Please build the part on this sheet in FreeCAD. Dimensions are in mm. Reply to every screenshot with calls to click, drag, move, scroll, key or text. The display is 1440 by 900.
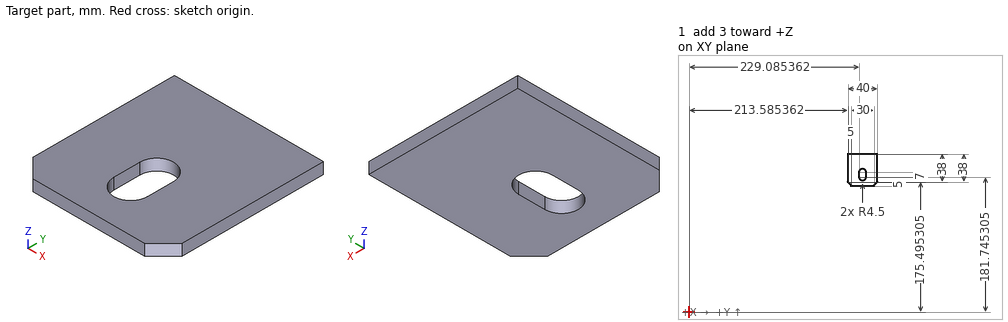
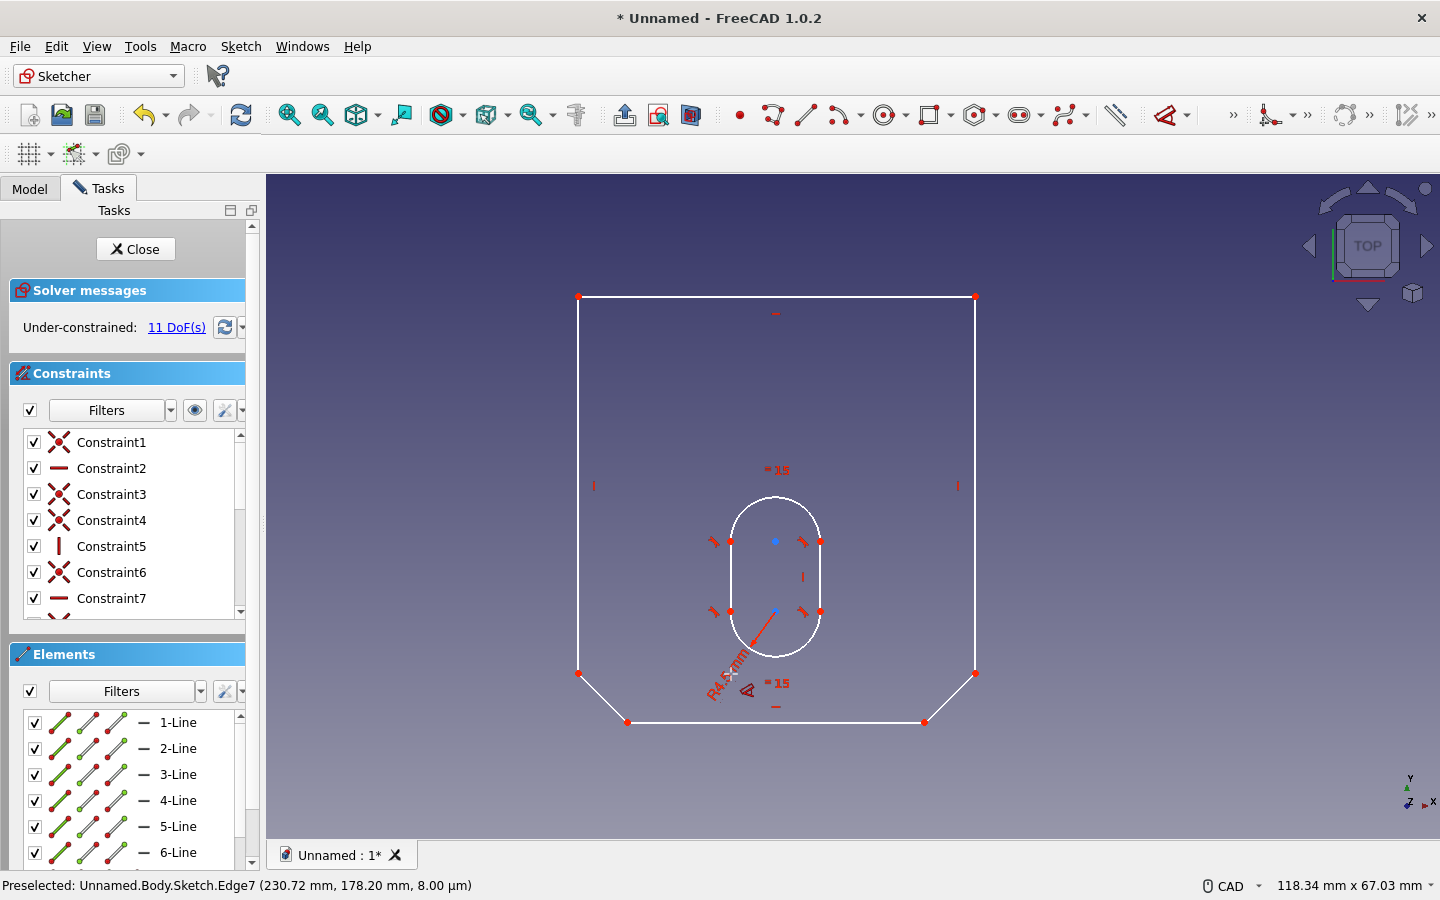
click(731, 591)
click(697, 577)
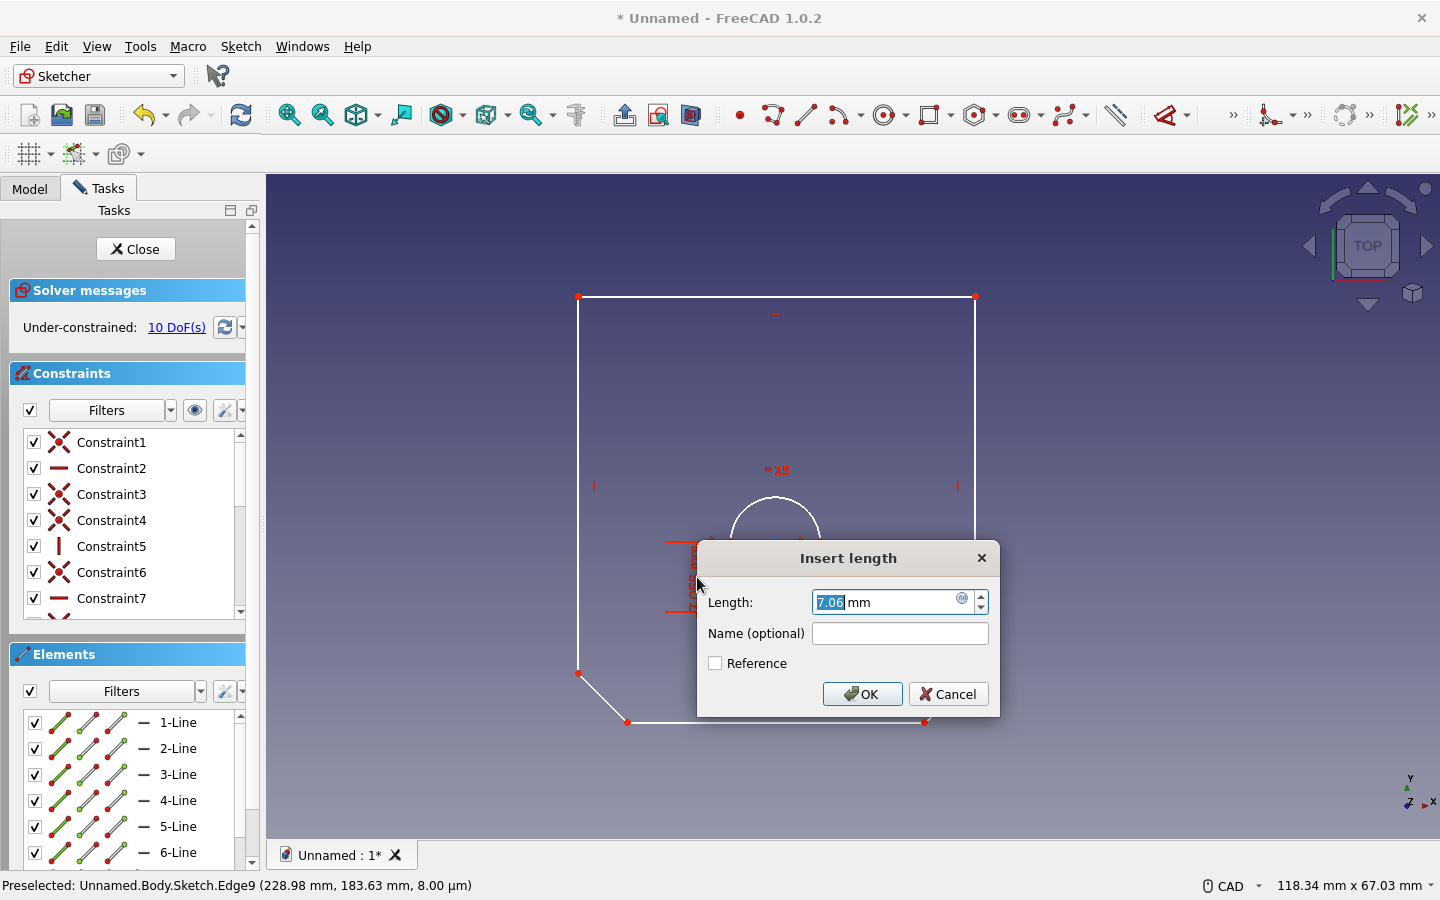
text(7)
key(Return)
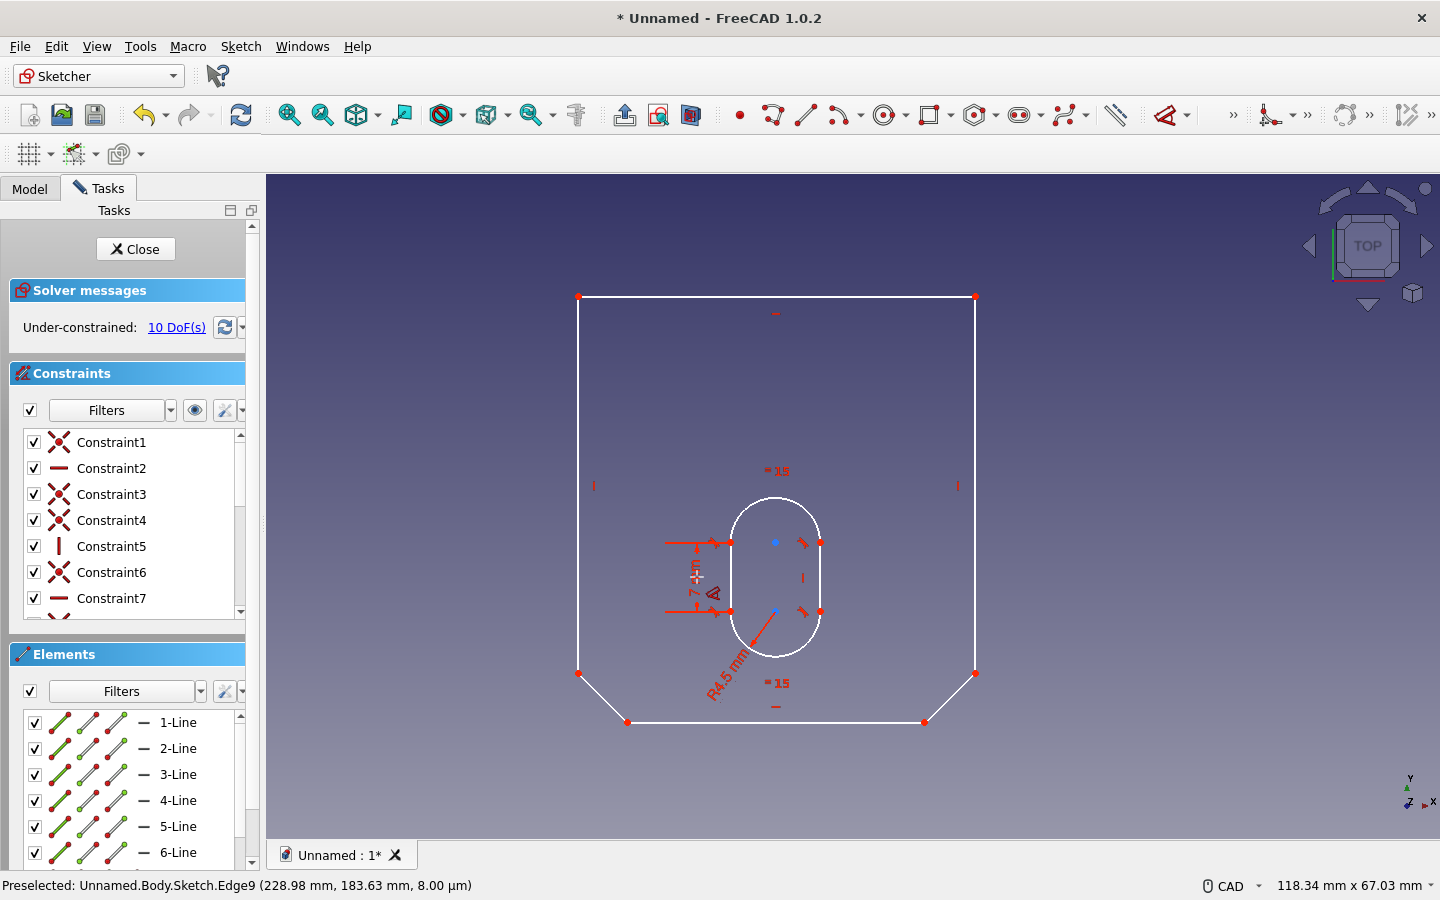
click(717, 723)
click(776, 757)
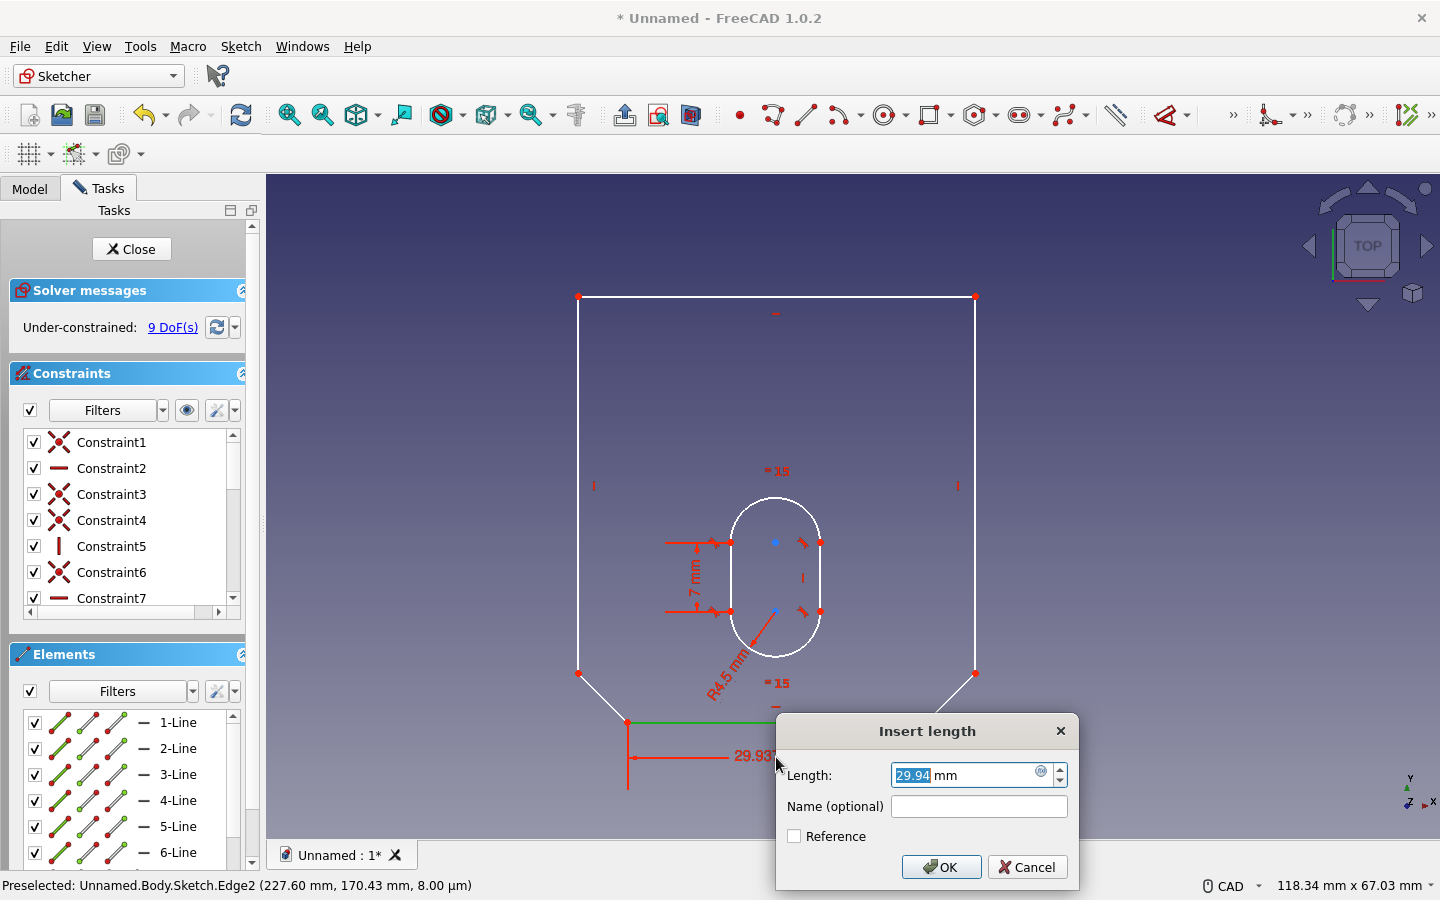
text(30)
key(Return)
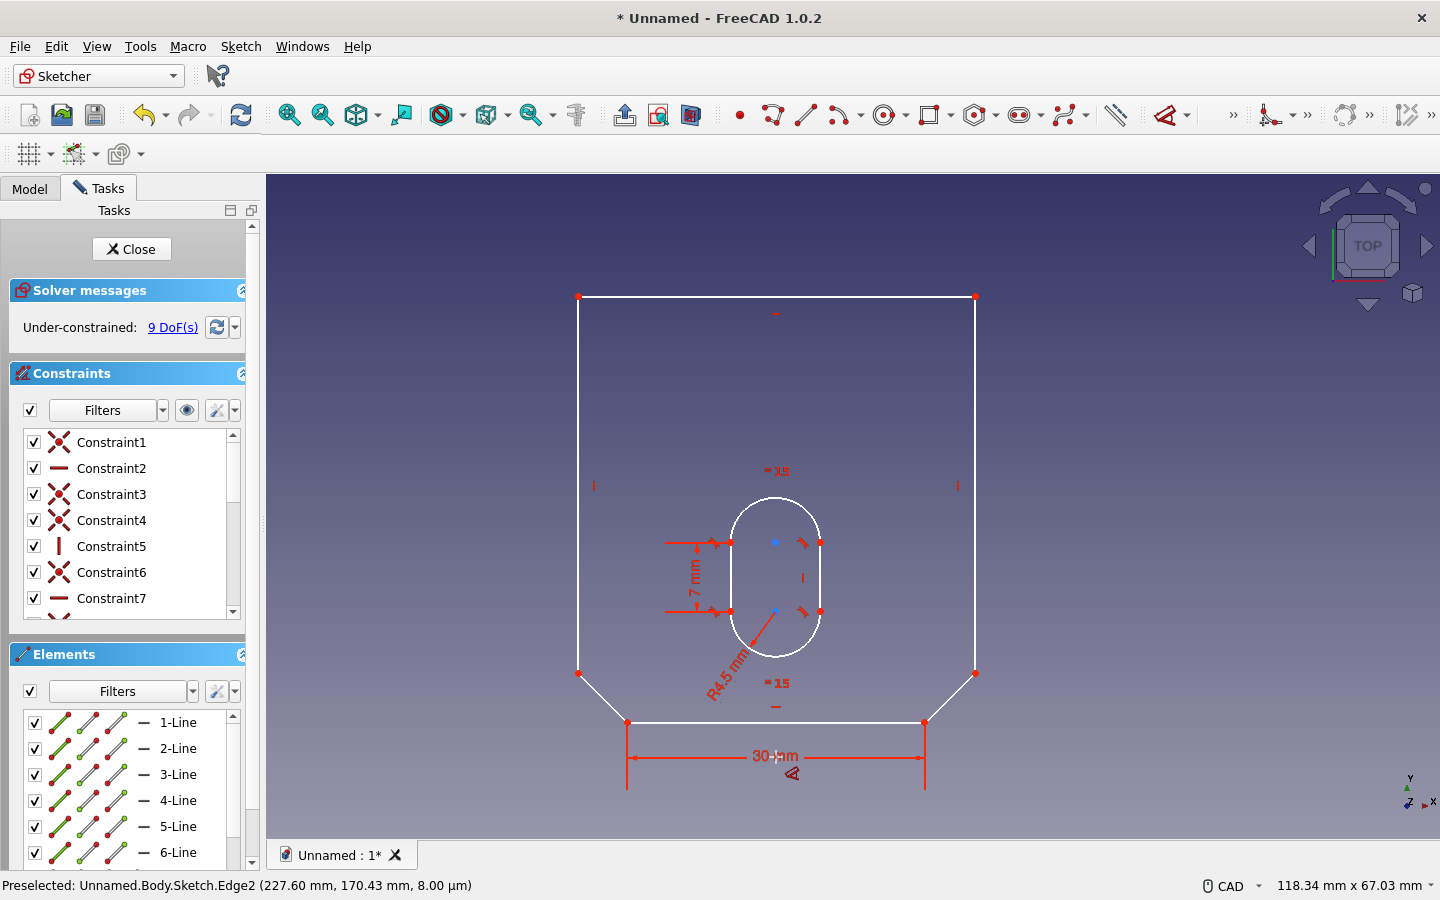
click(975, 561)
click(1009, 486)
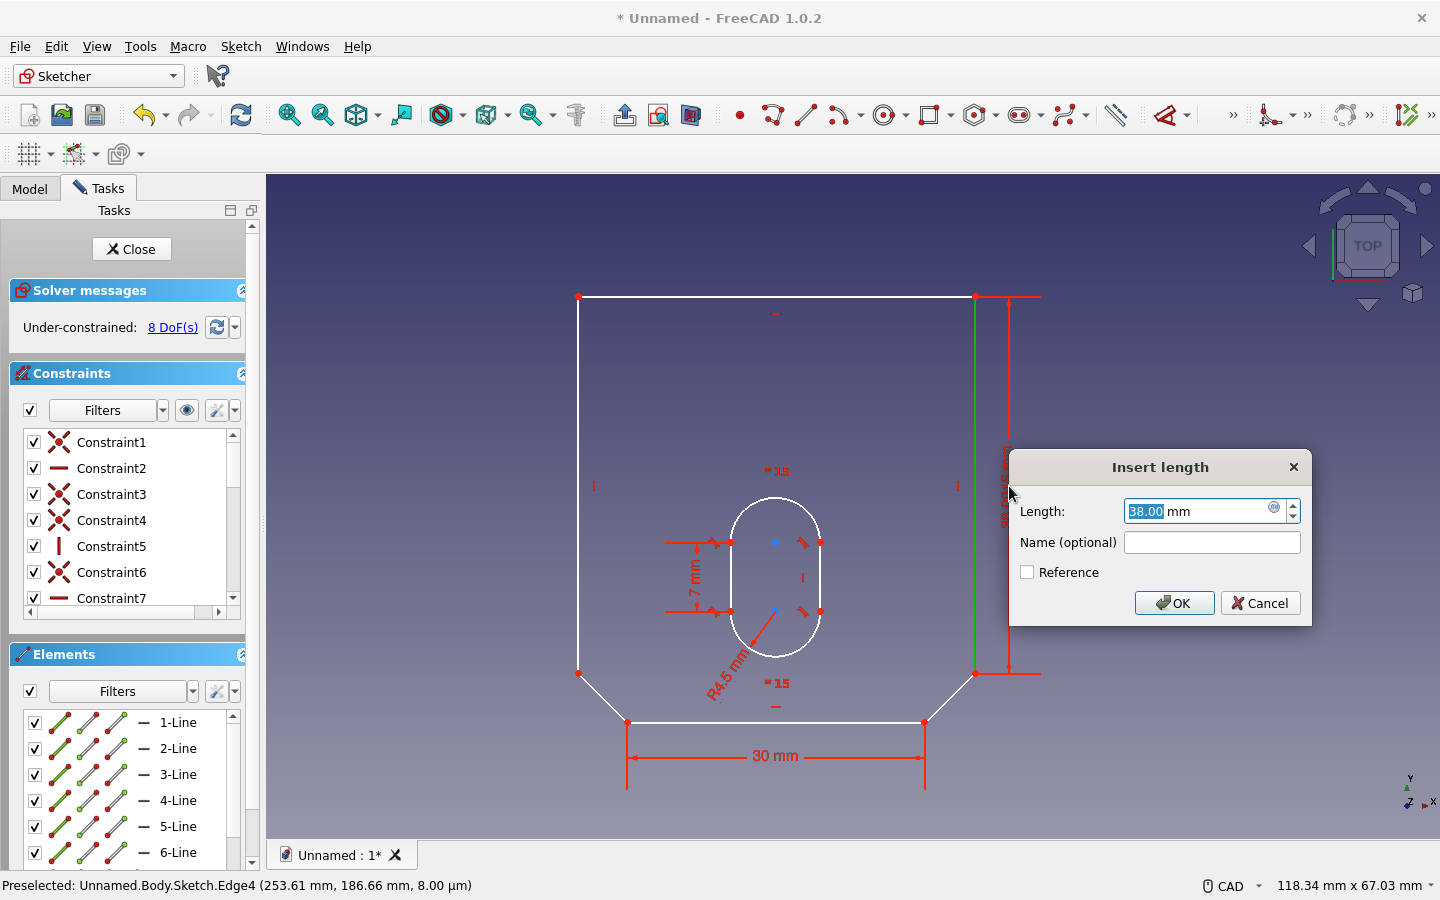
text(38)
key(Return)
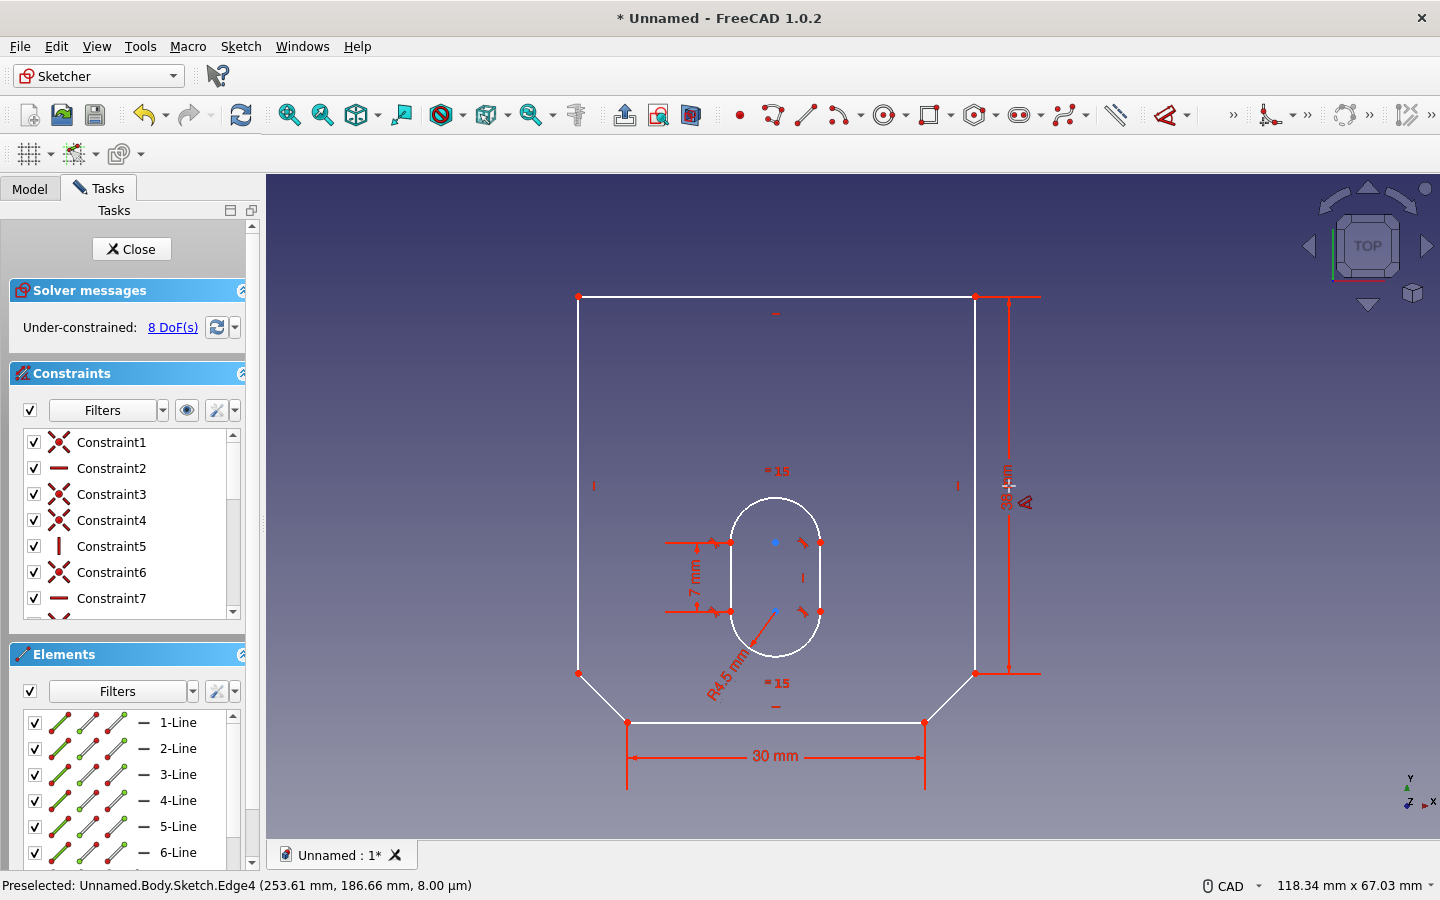
click(856, 297)
click(777, 263)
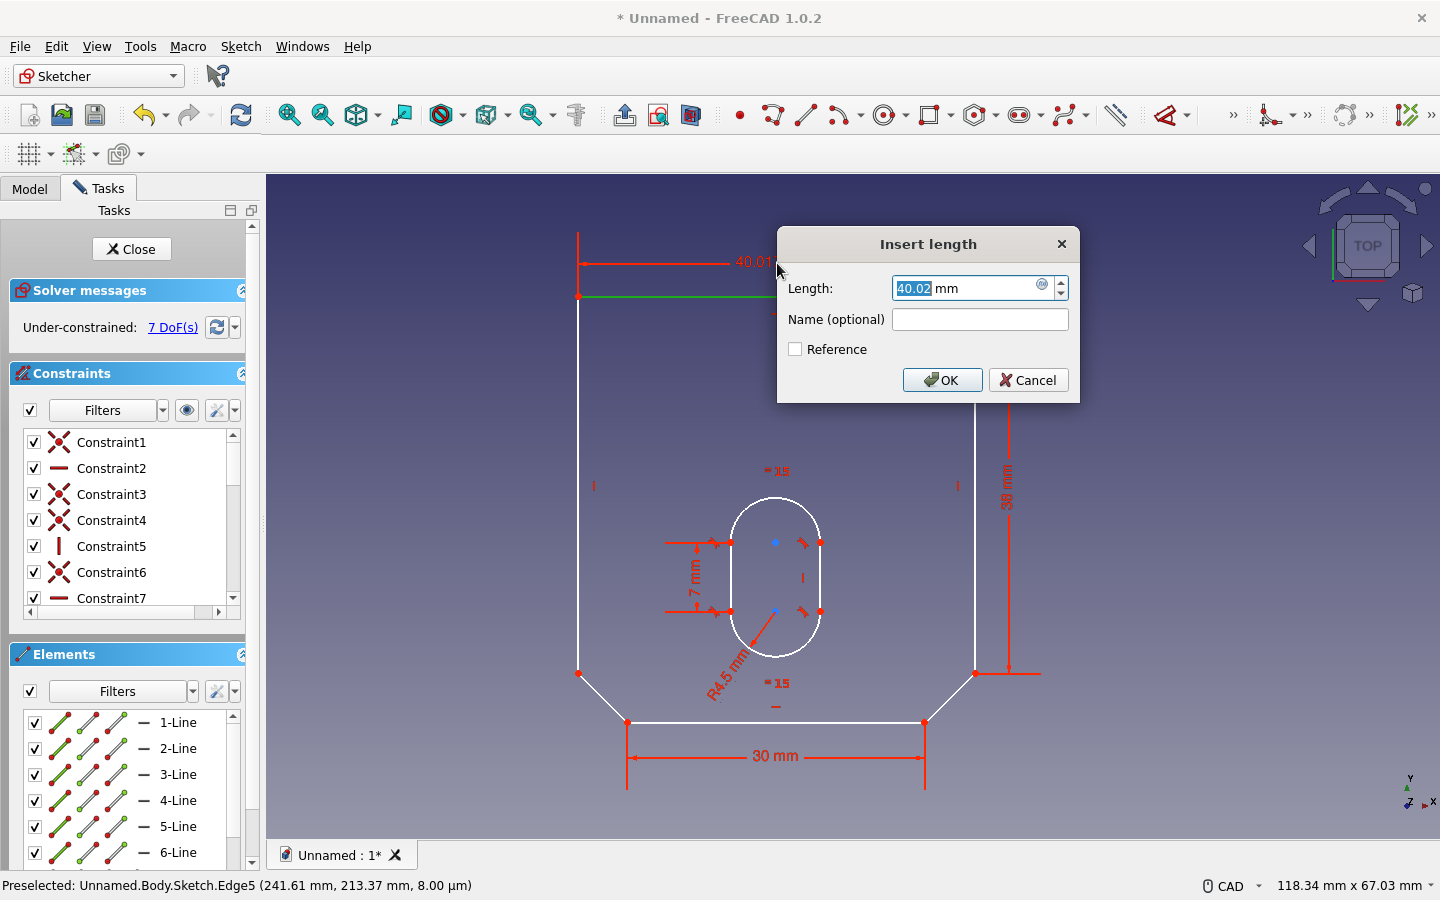
text(40)
key(Return)